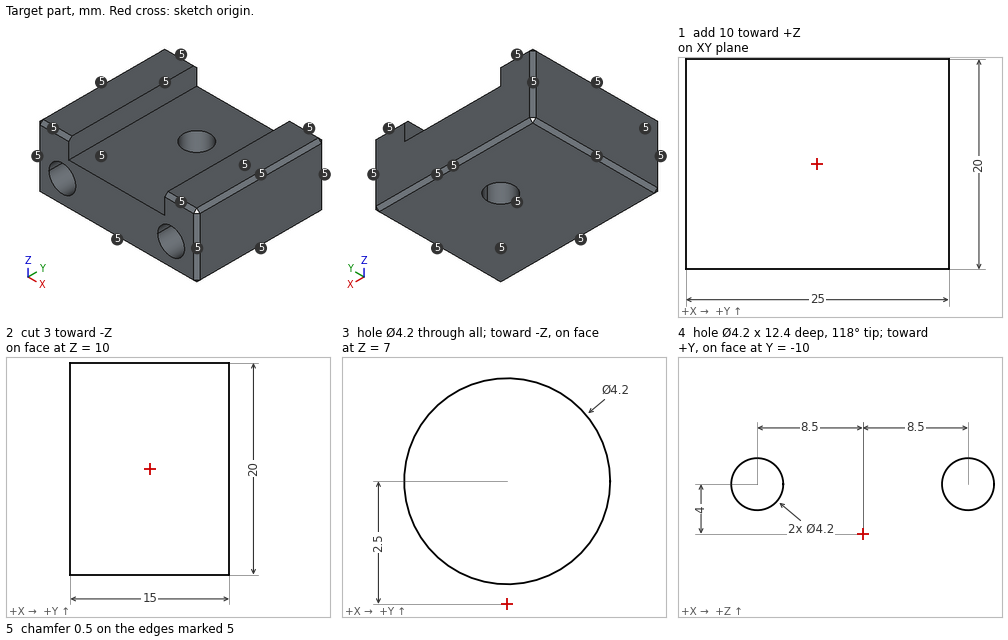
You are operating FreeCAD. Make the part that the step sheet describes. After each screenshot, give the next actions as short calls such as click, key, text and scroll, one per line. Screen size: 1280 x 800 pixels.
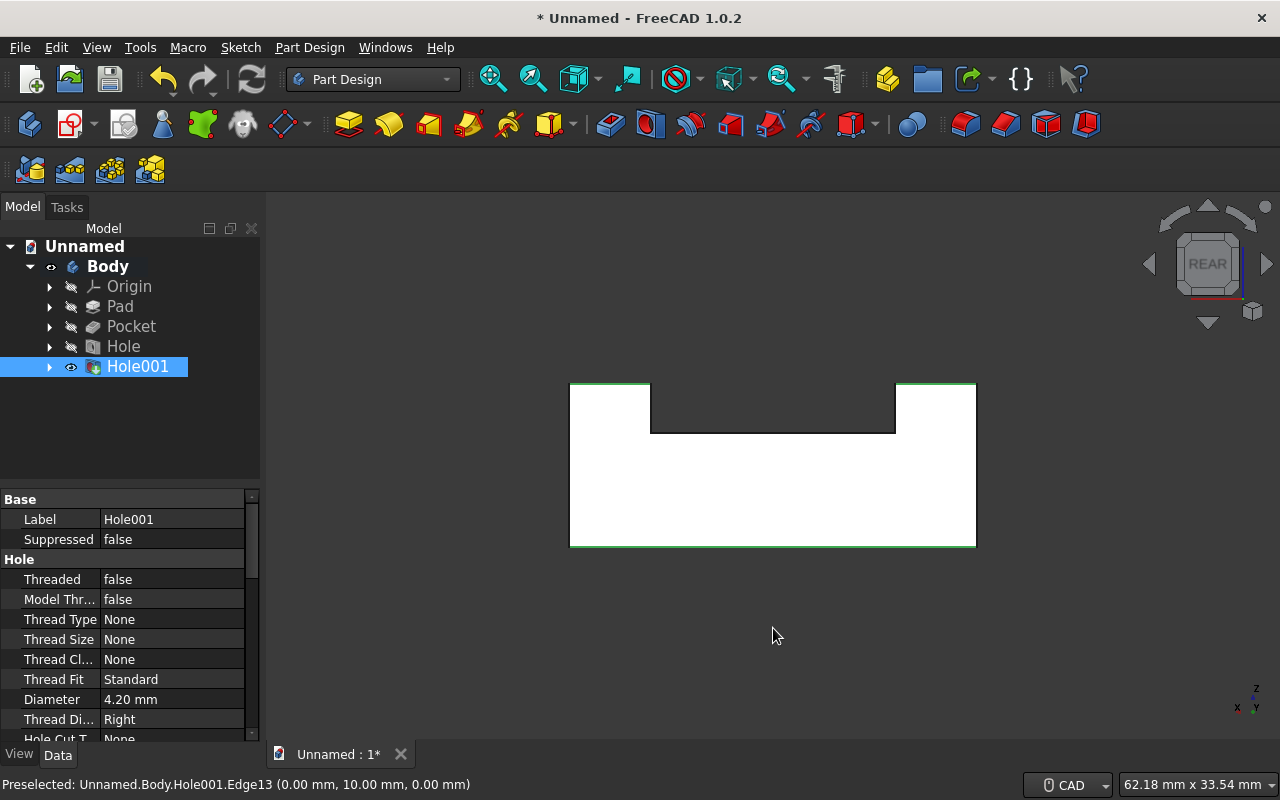
key(v)
key(f)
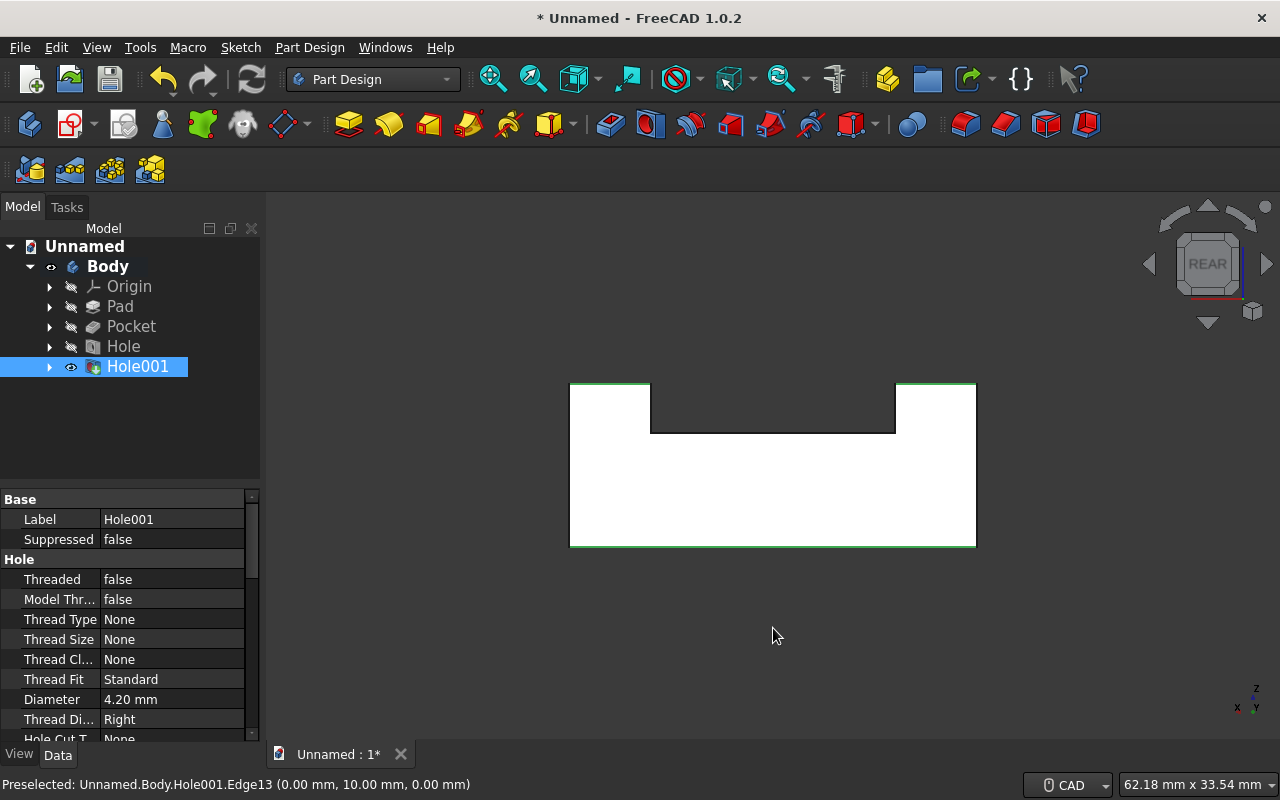
key(6)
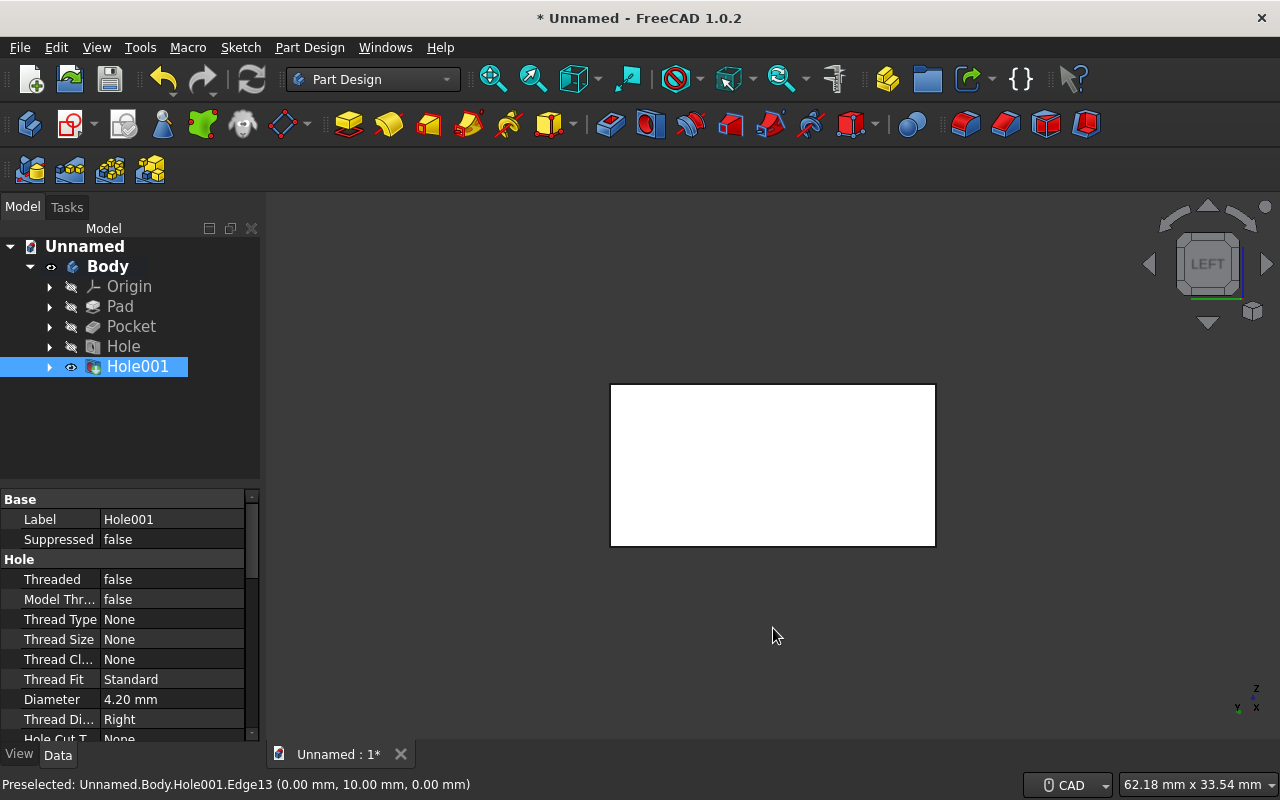
click(494, 80)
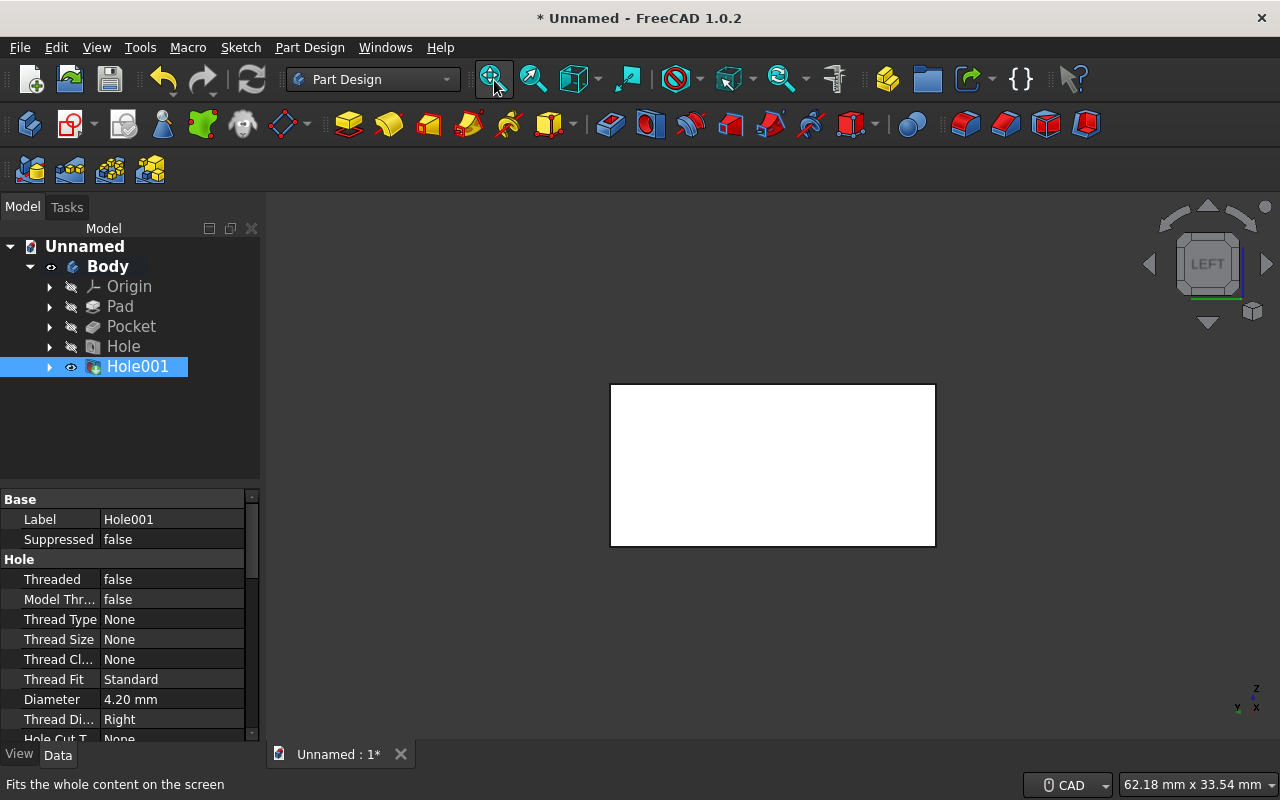
click(726, 464, ctrl)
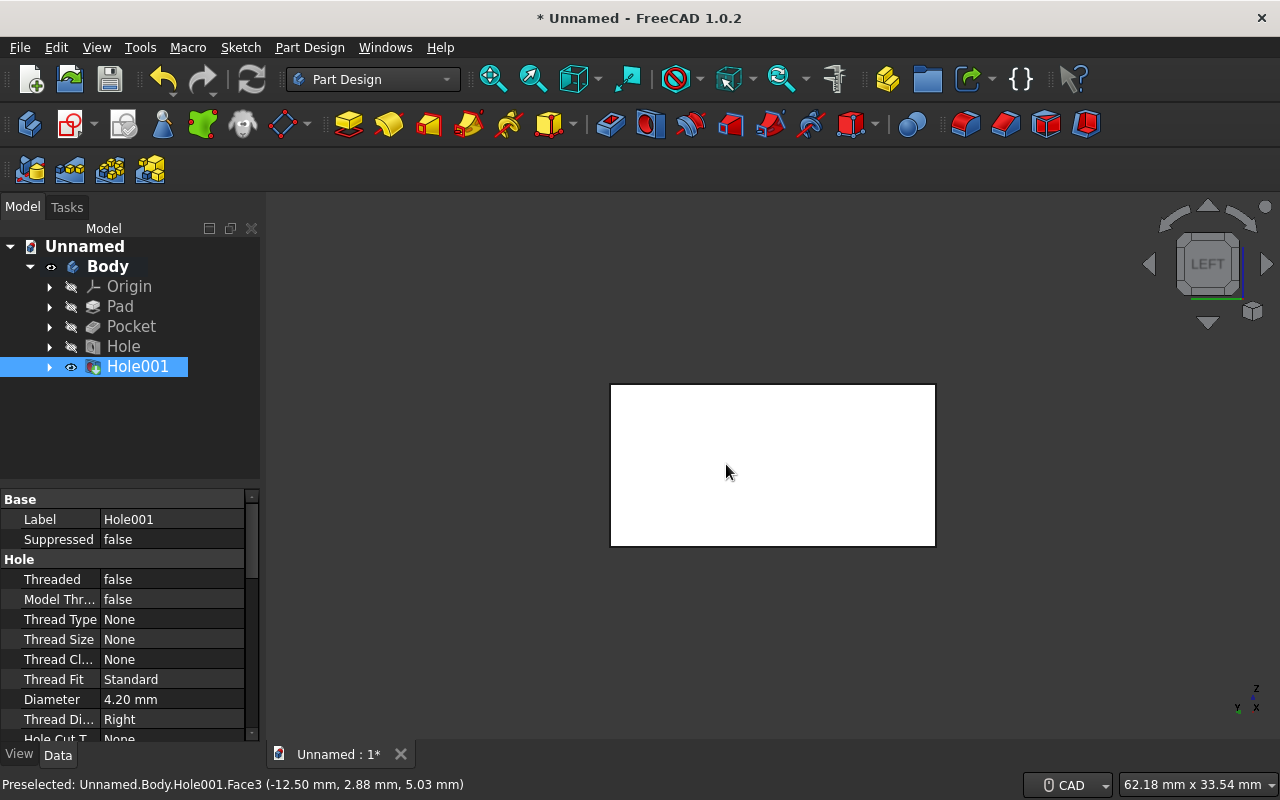
click(1006, 124)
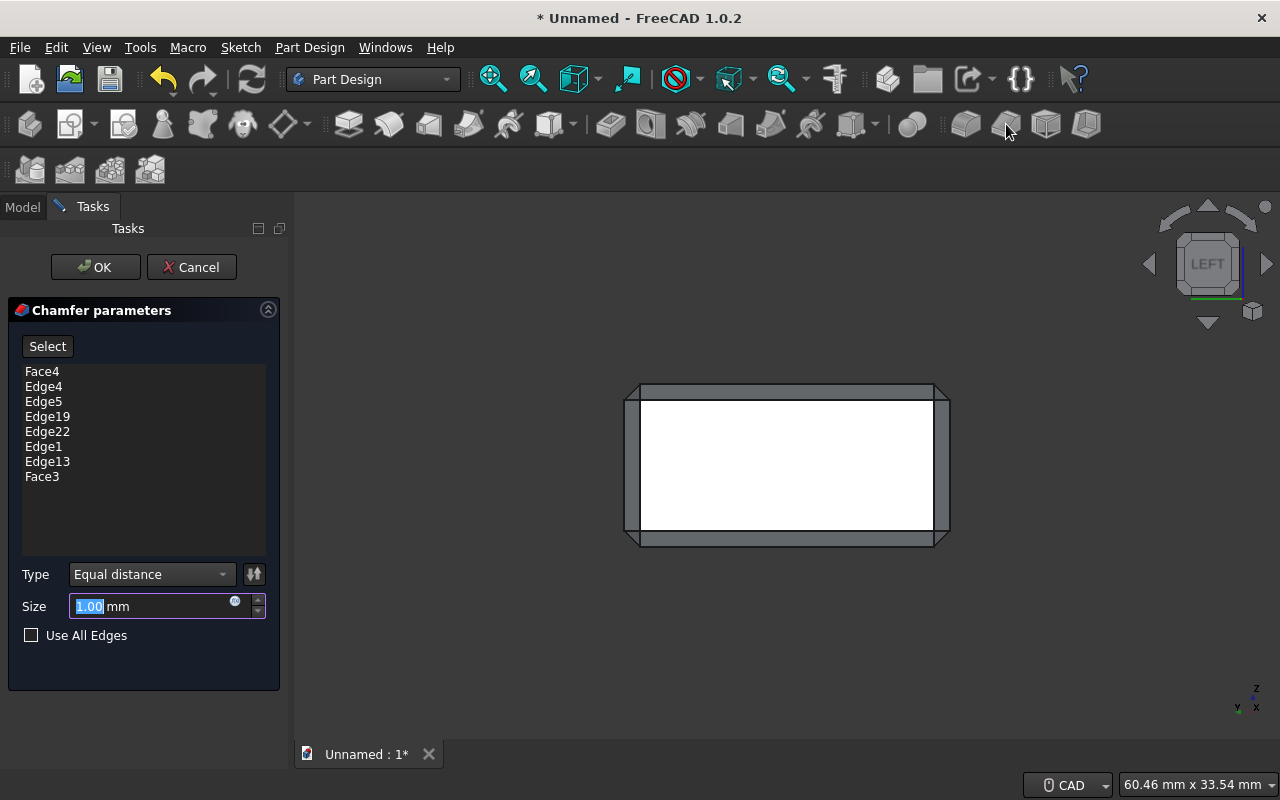
text(0.5)
key(Tab)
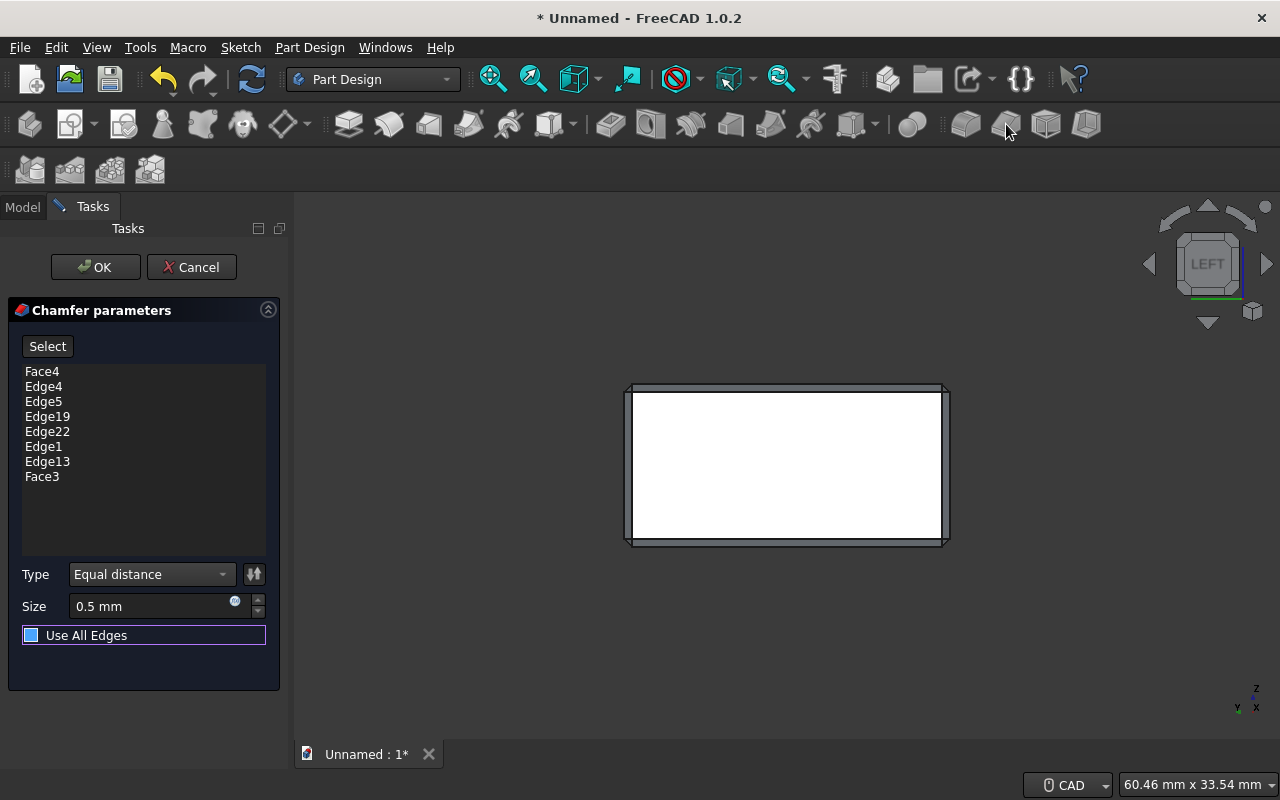
click(96, 267)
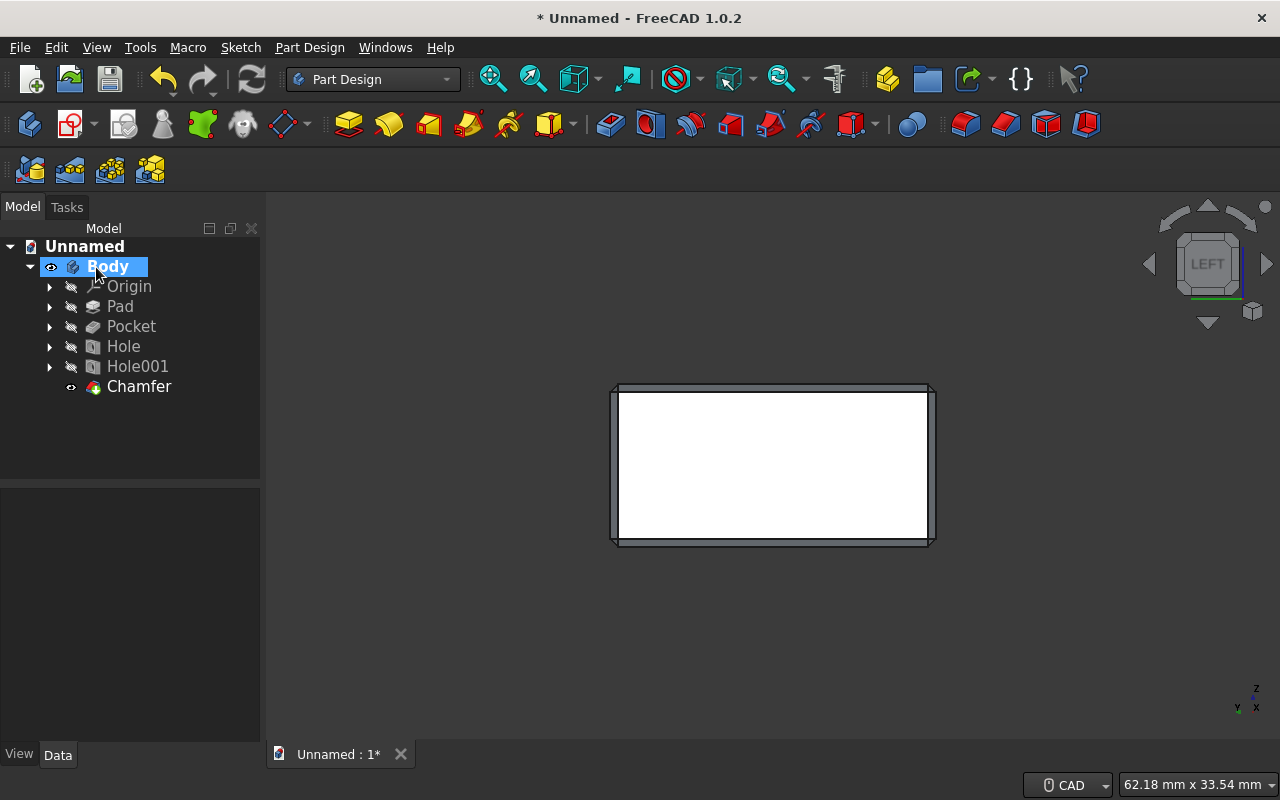
key(0)